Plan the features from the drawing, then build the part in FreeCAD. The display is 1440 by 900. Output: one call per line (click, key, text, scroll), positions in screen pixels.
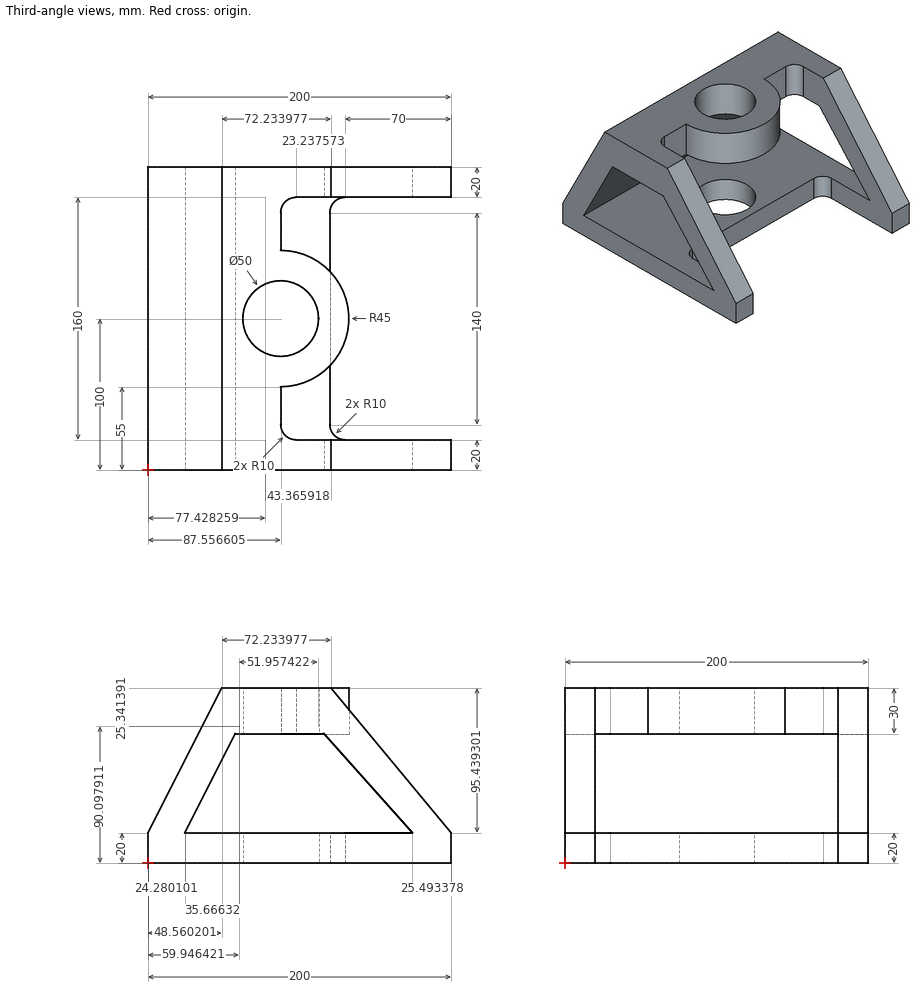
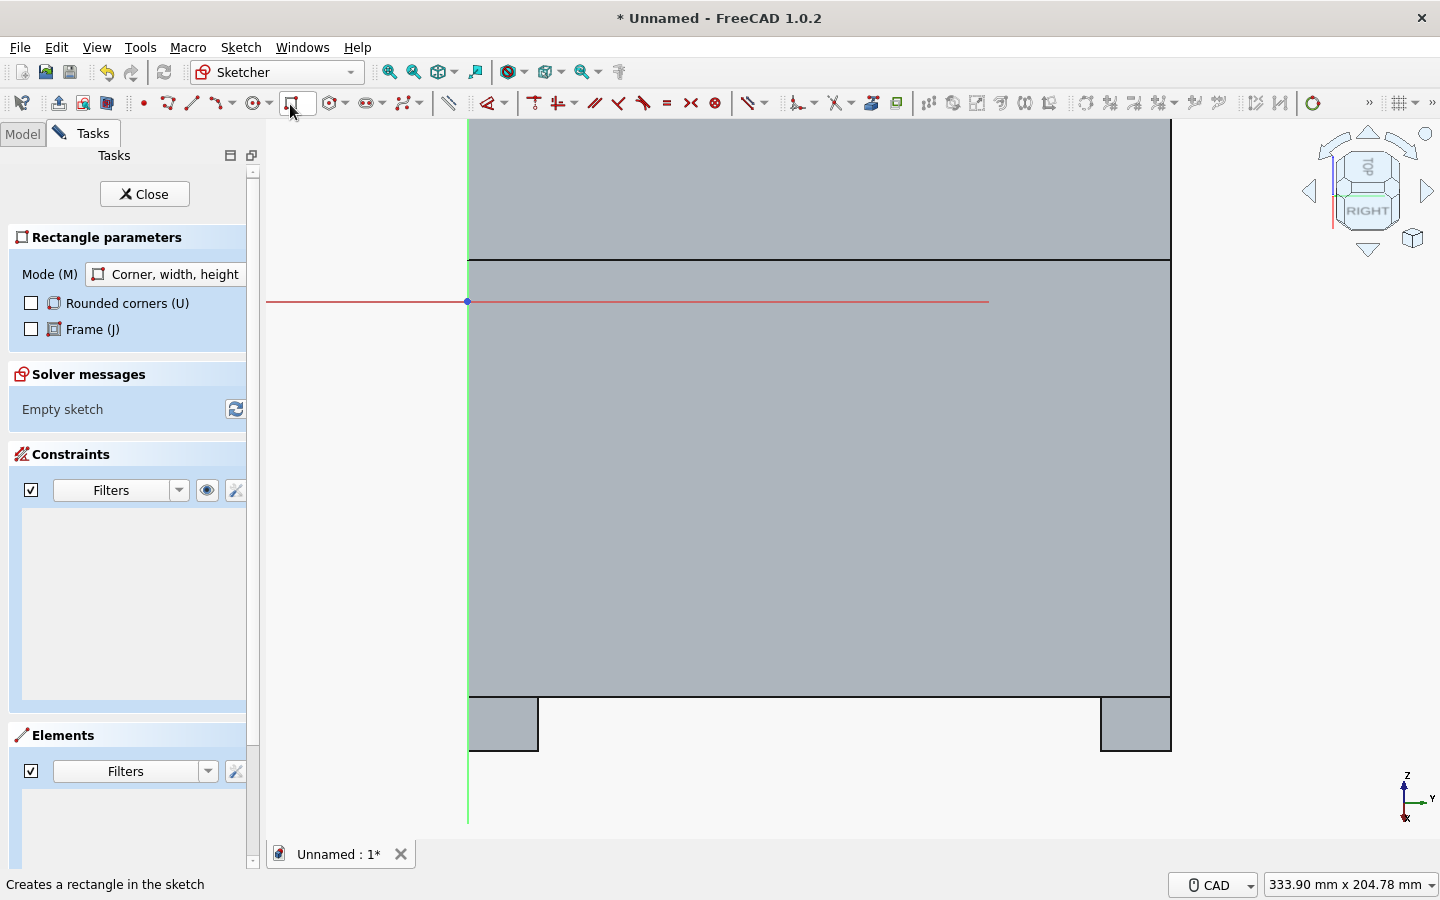
click(538, 260)
click(1101, 697)
key(Escape)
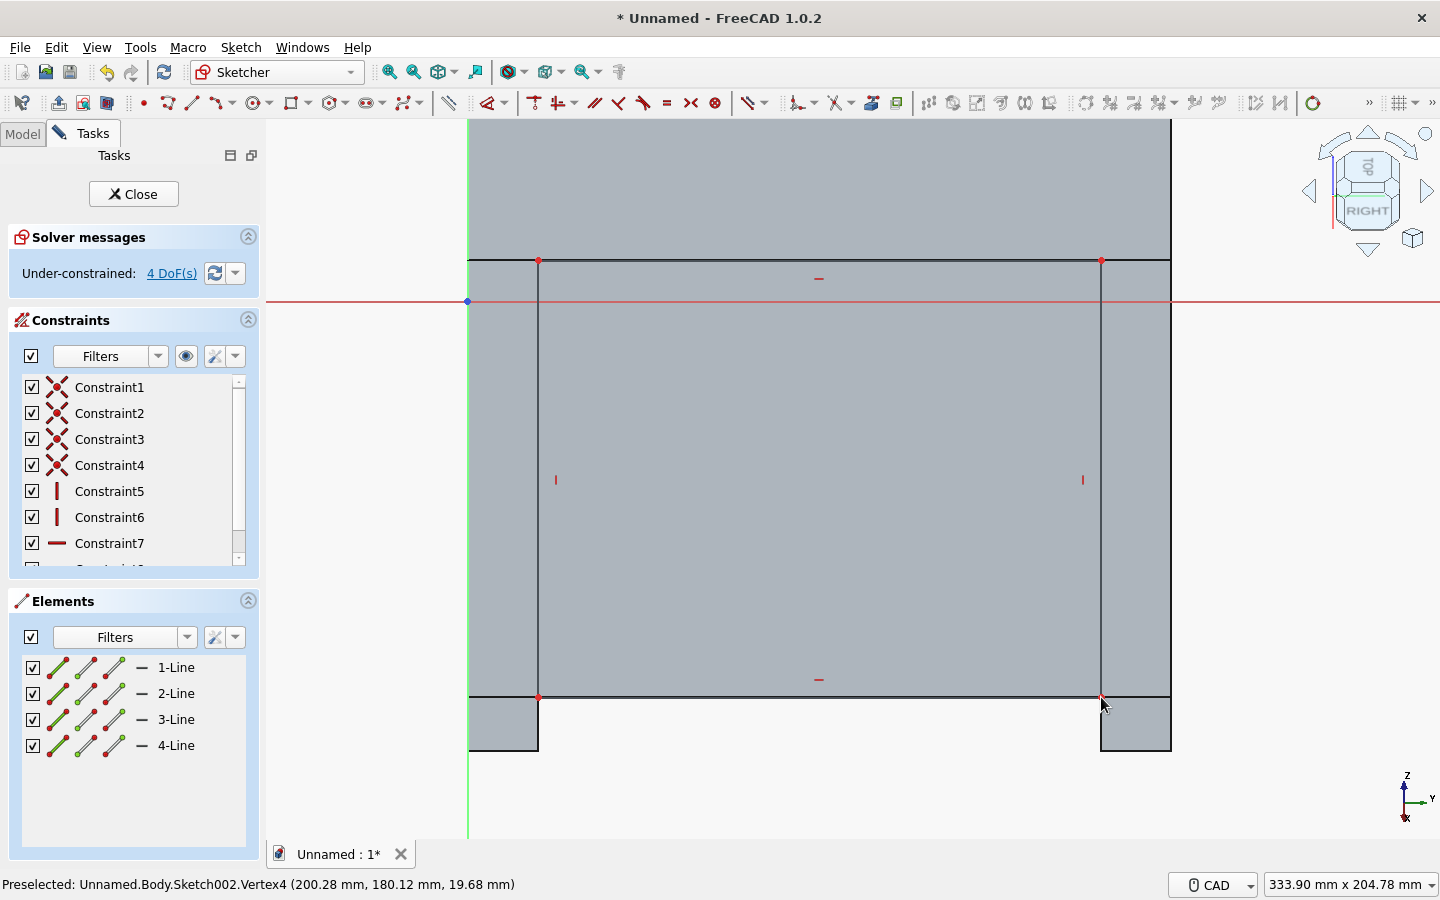
click(488, 104)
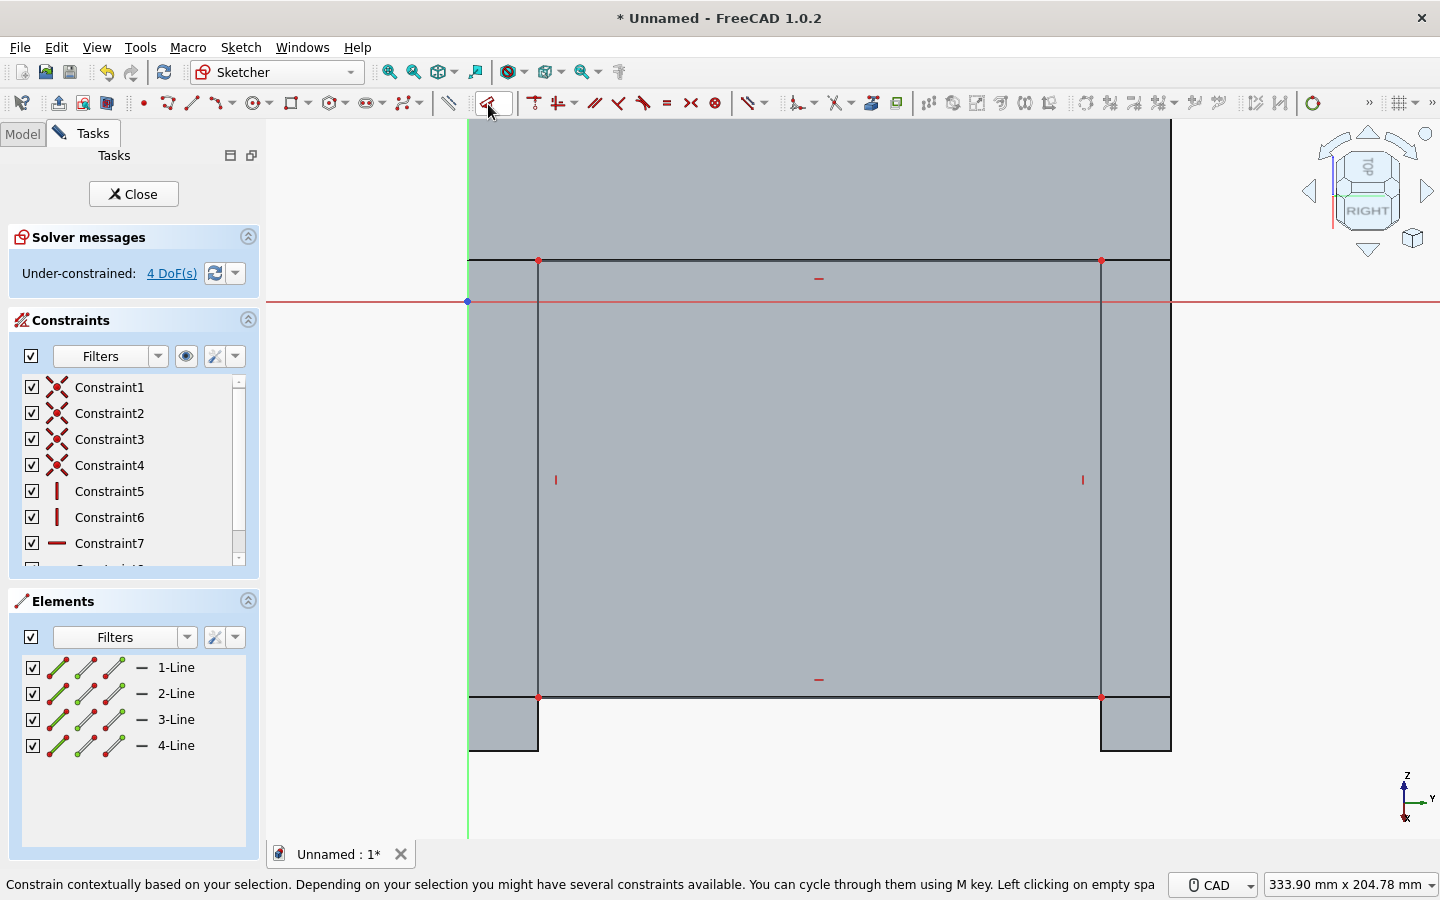
click(707, 698)
click(819, 732)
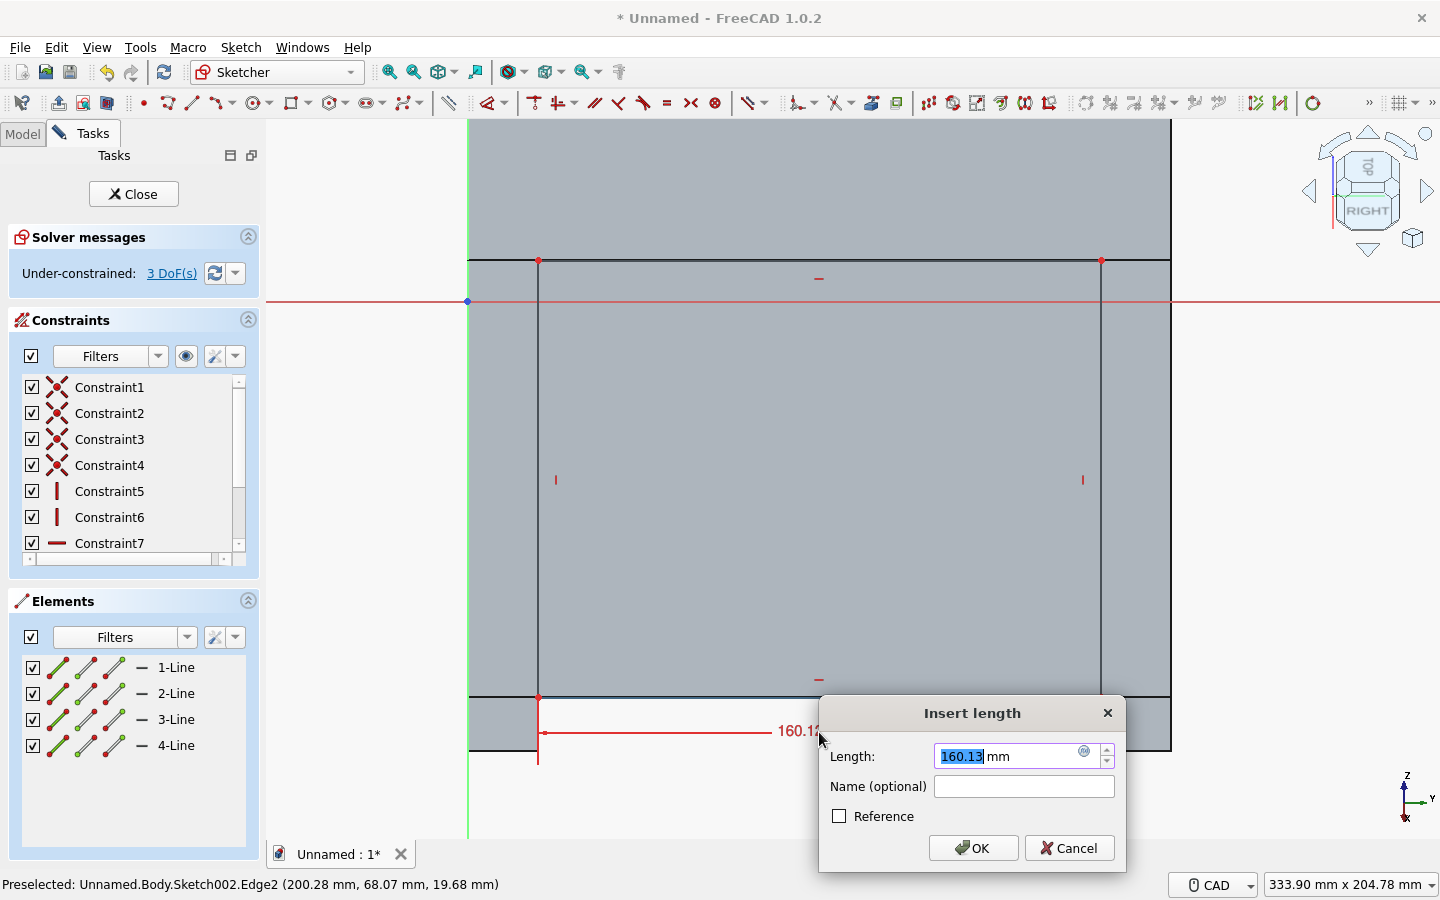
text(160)
key(Return)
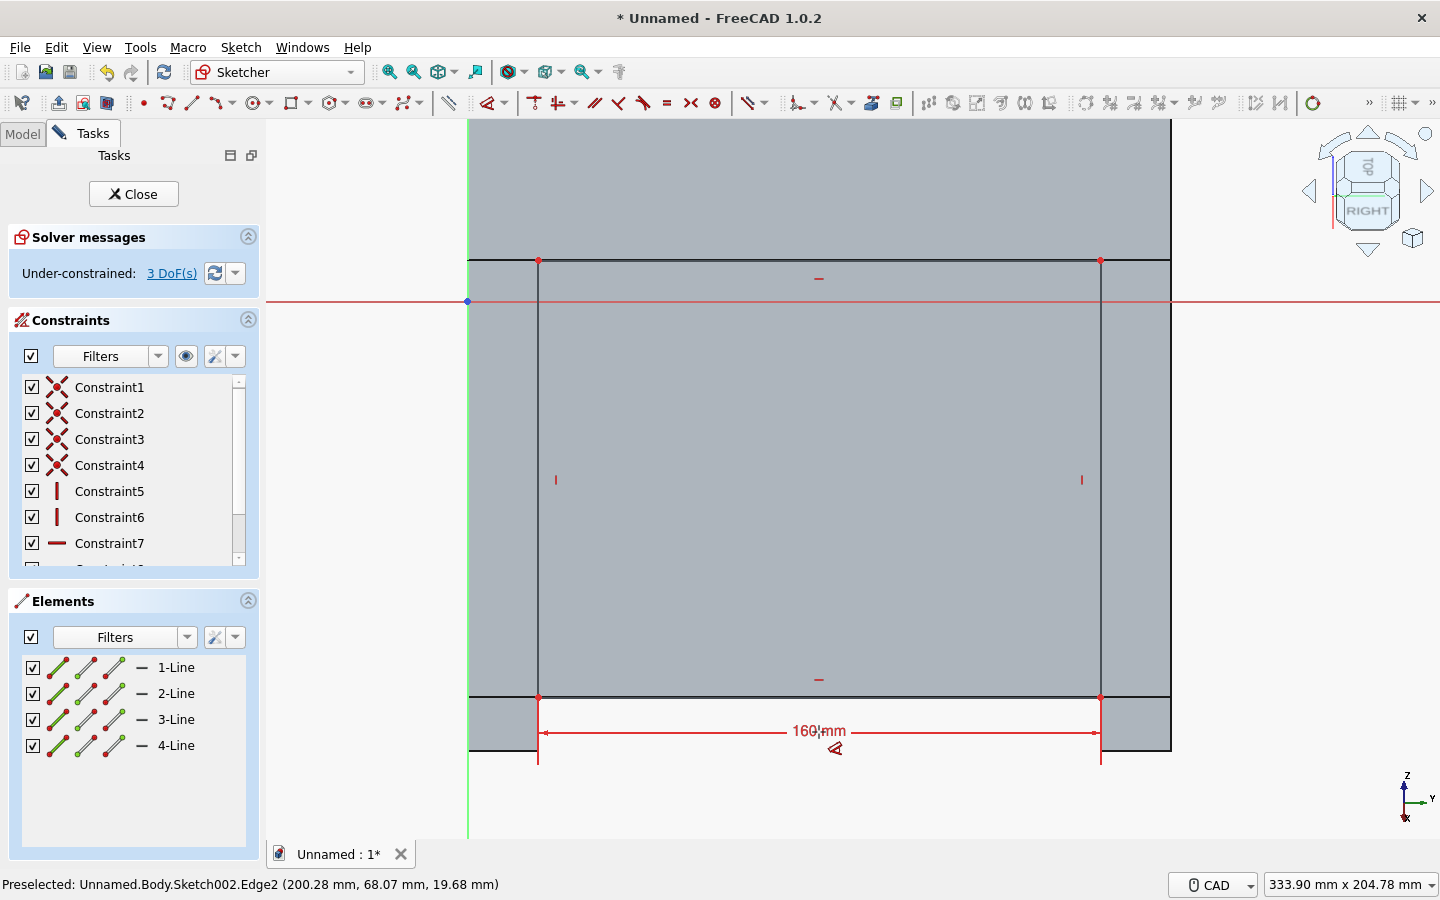
click(538, 261)
click(503, 227)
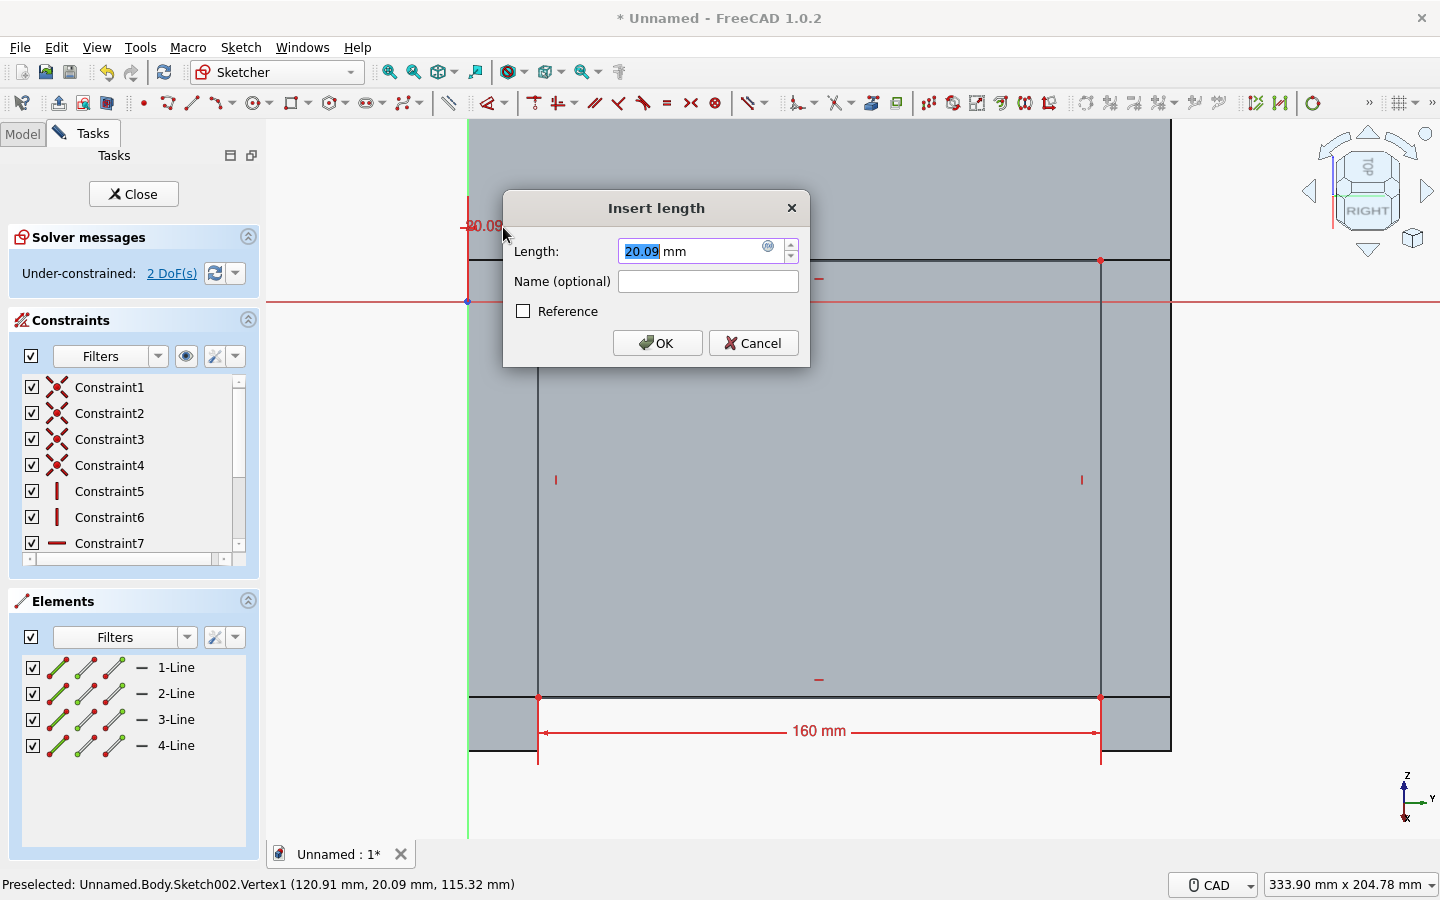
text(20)
key(Return)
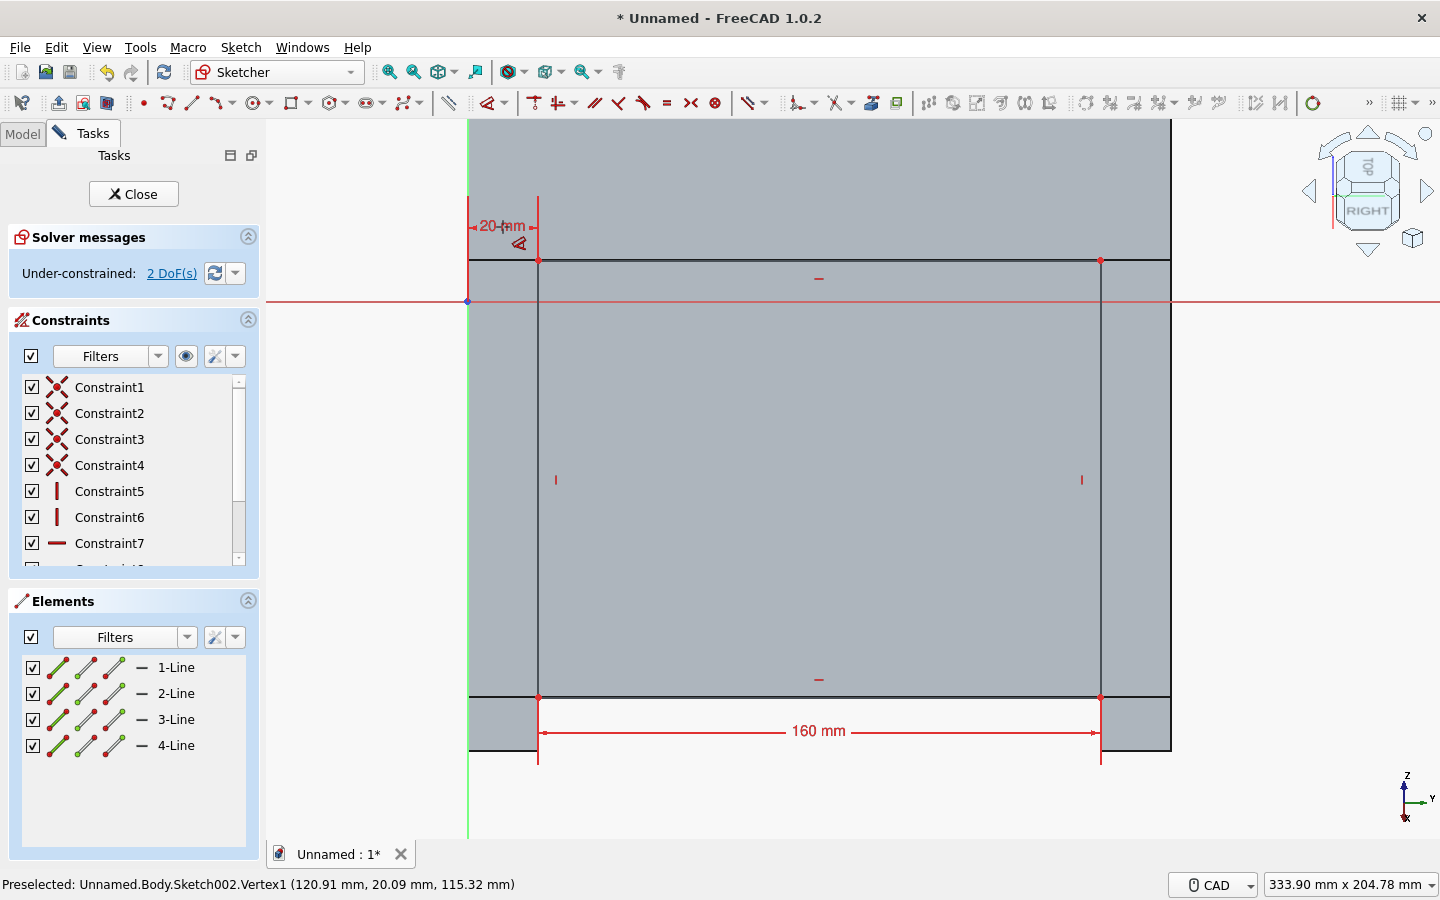
click(538, 392)
click(504, 480)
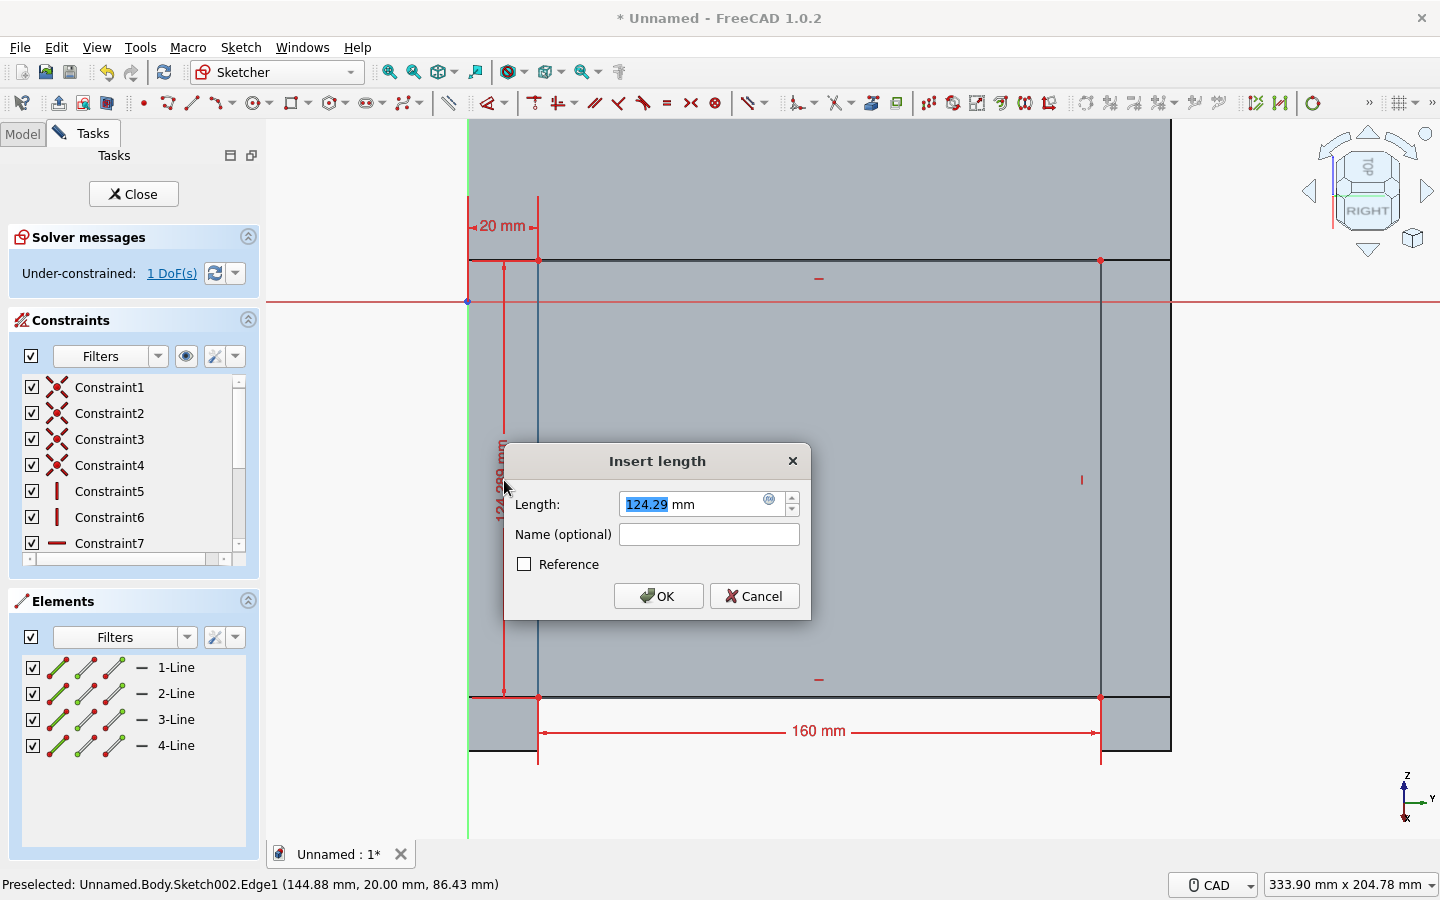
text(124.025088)
key(Return)